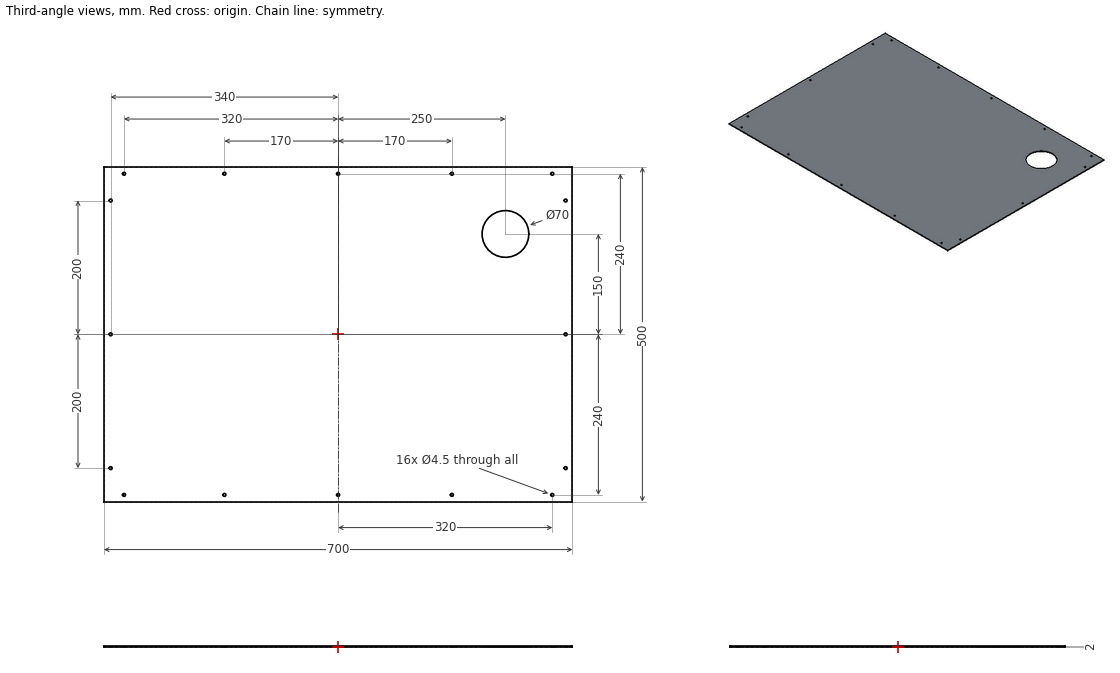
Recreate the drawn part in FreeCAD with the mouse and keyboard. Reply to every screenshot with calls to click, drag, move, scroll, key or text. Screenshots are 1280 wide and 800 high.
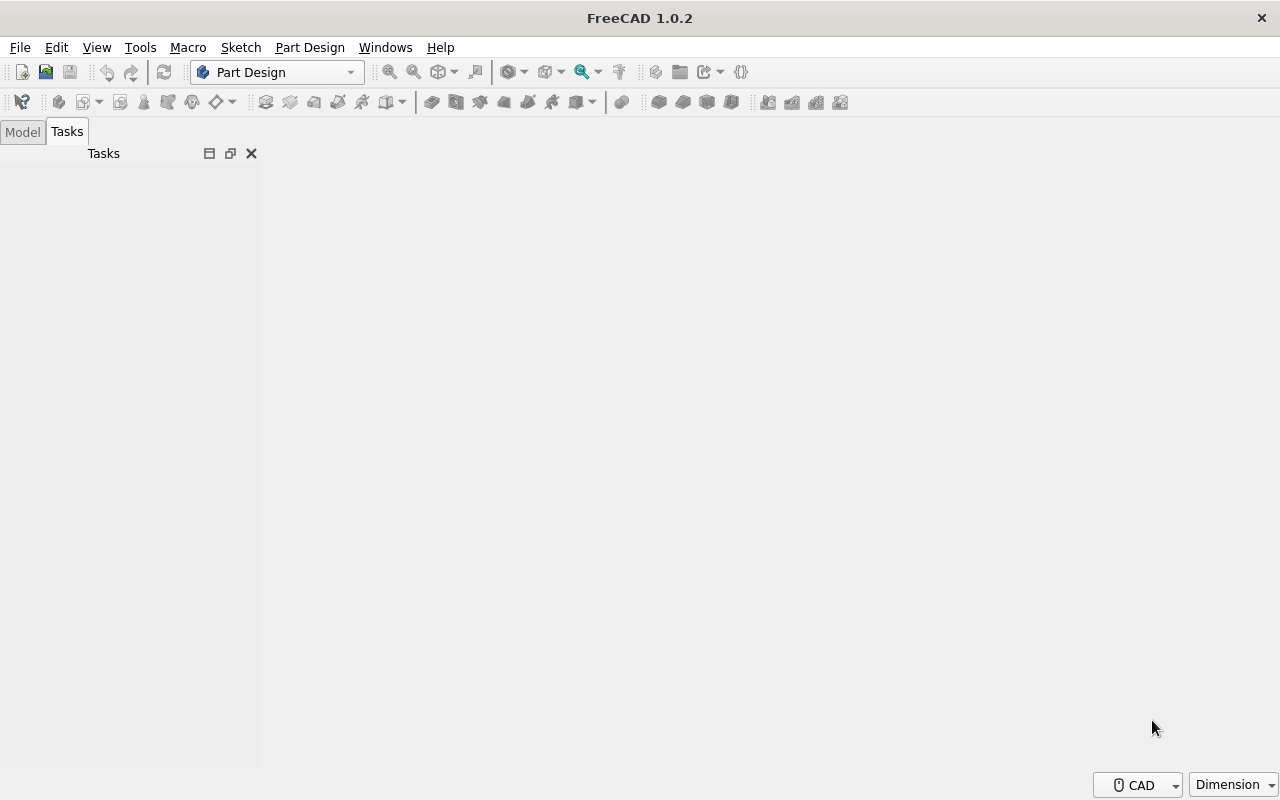
key(ctrl+n)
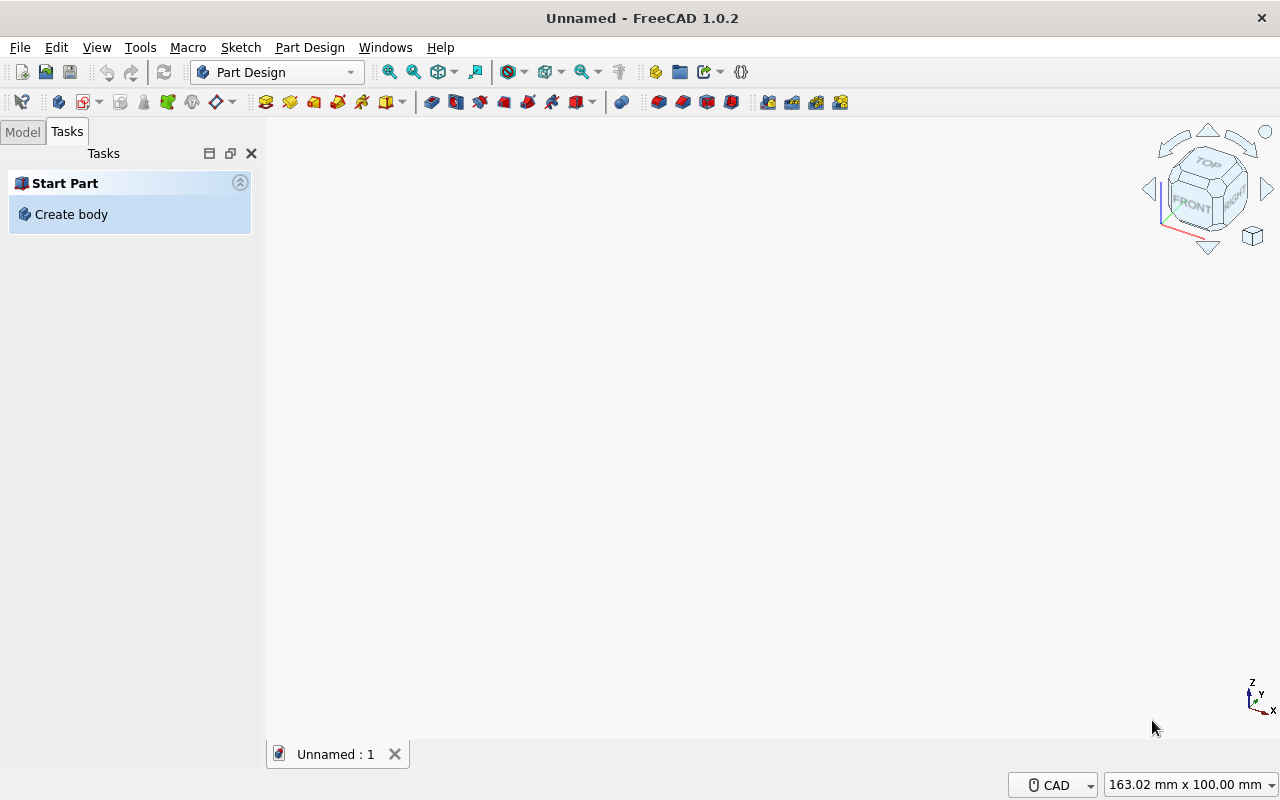
click(84, 102)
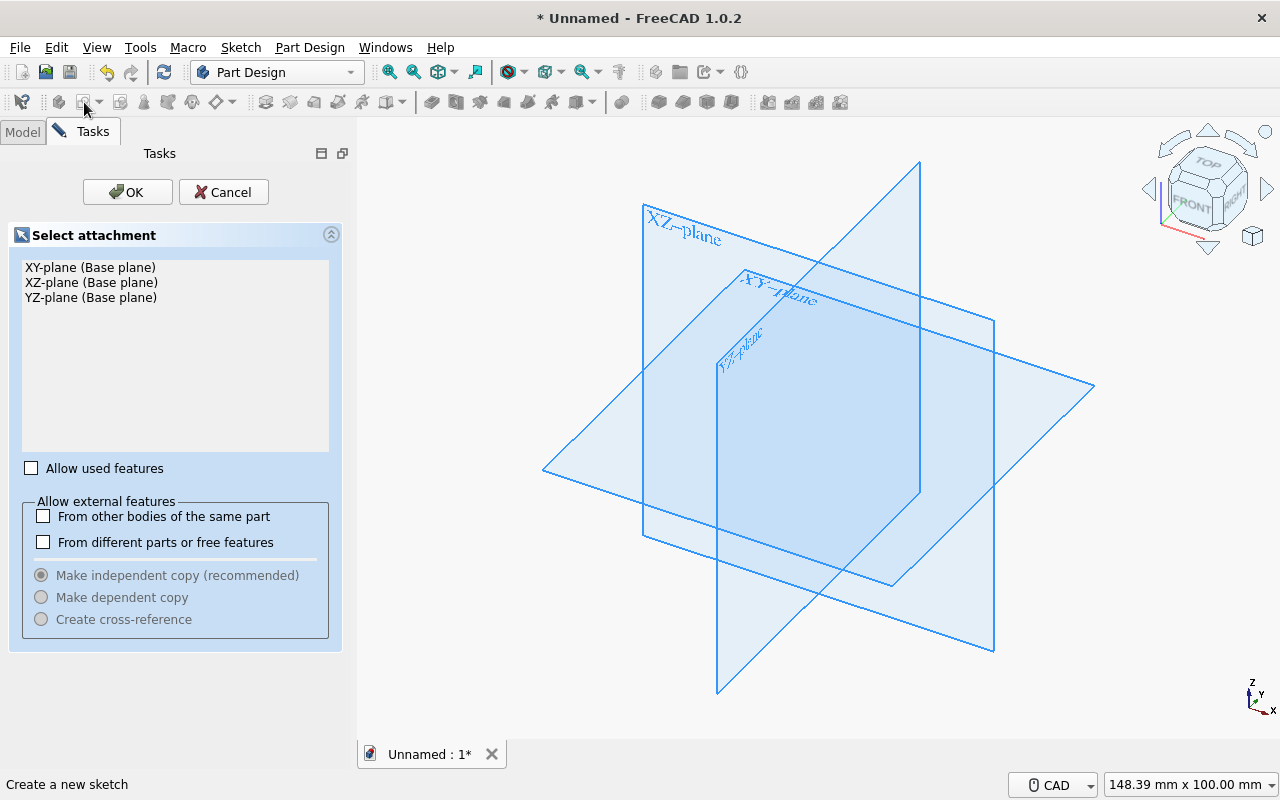
click(82, 268)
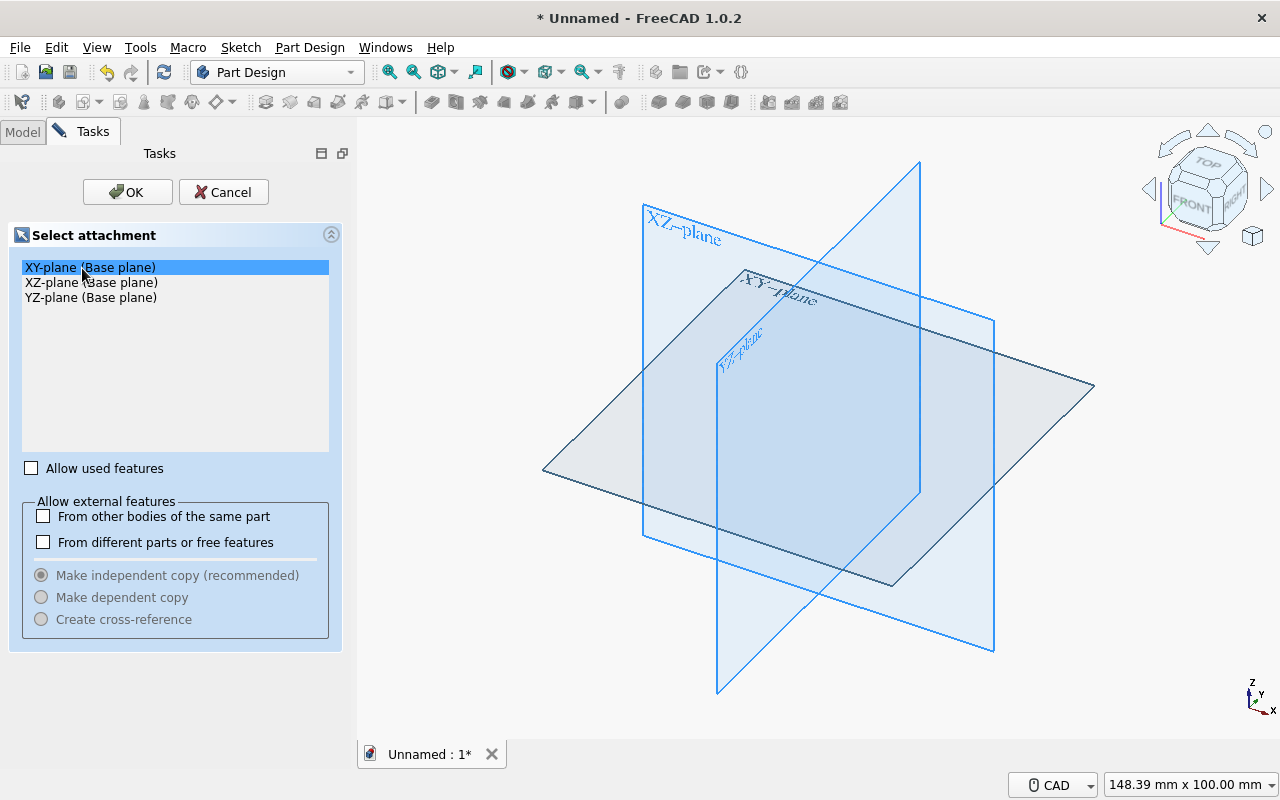
click(128, 192)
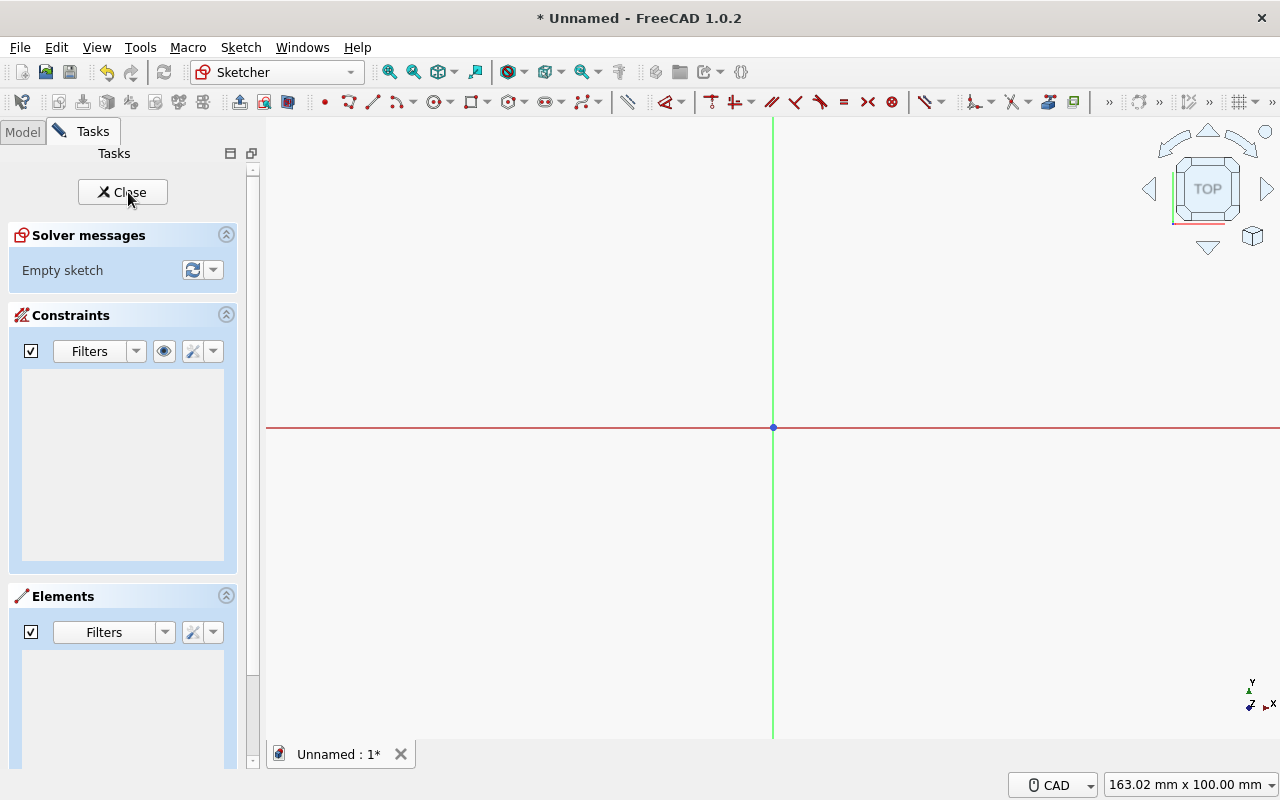
scroll(694, 428, down, 10)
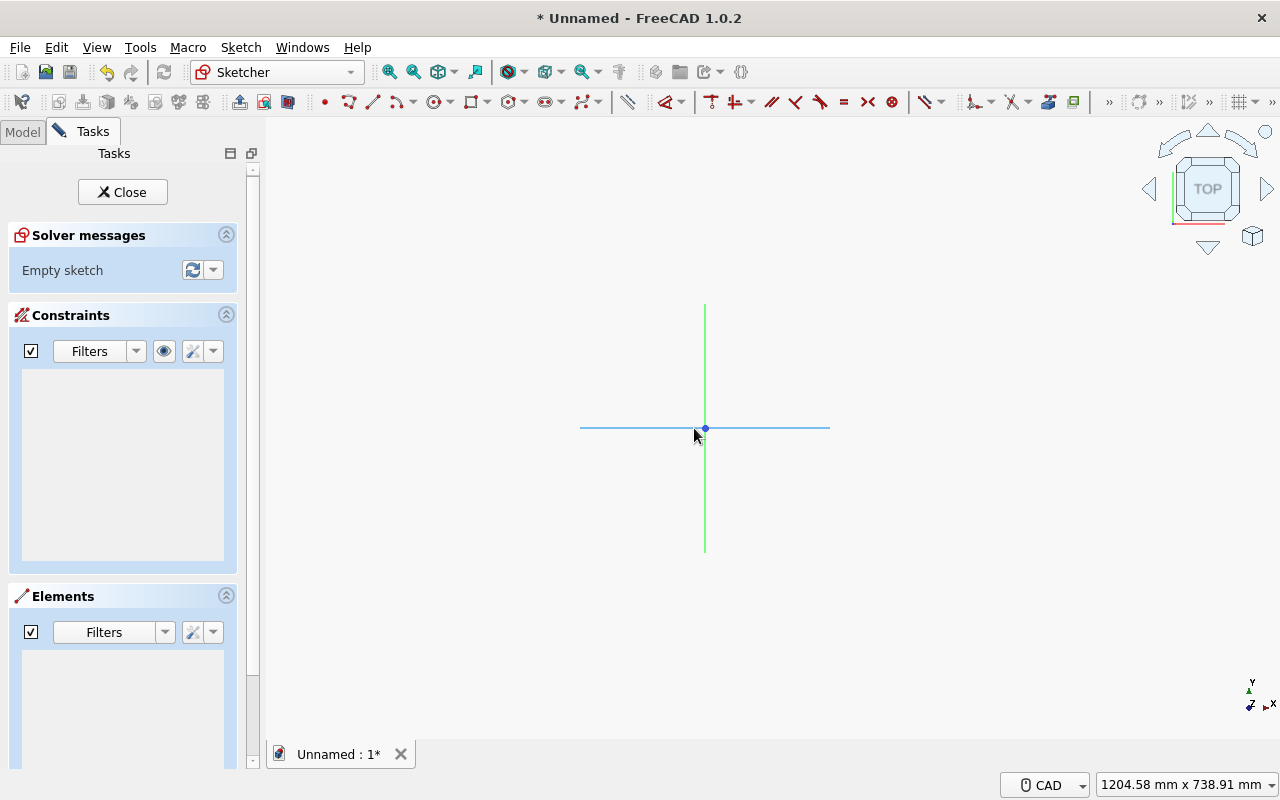
key(g)
key(v)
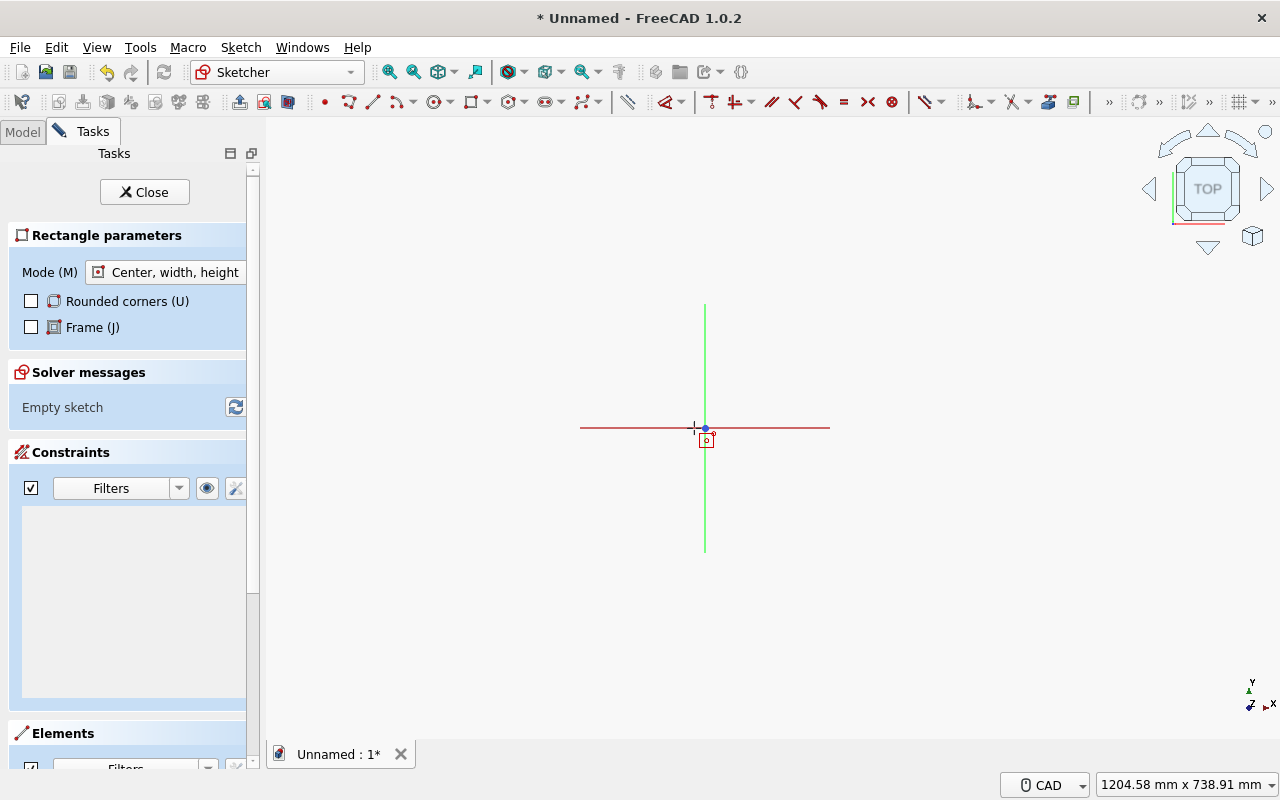
click(705, 428)
move(1000, 218)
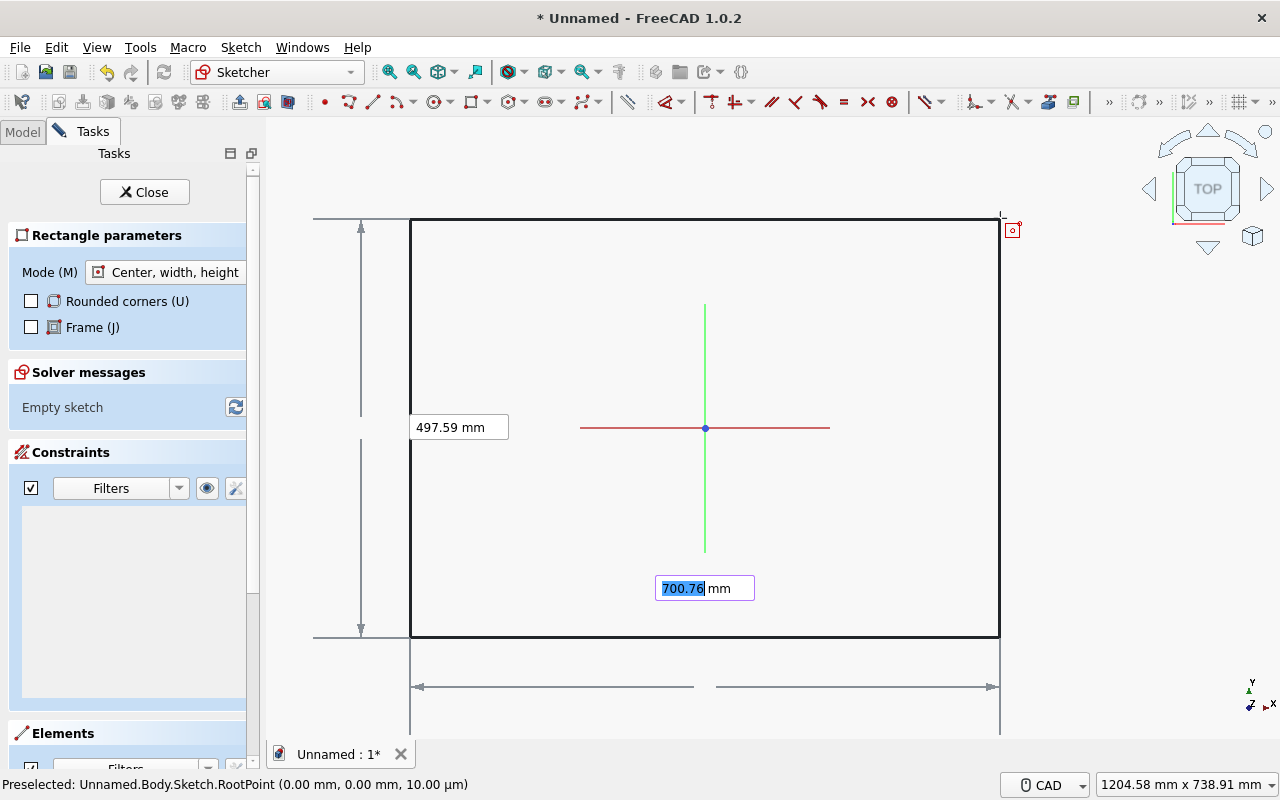
text(700)
key(Tab)
text(500)
key(Return)
key(Escape)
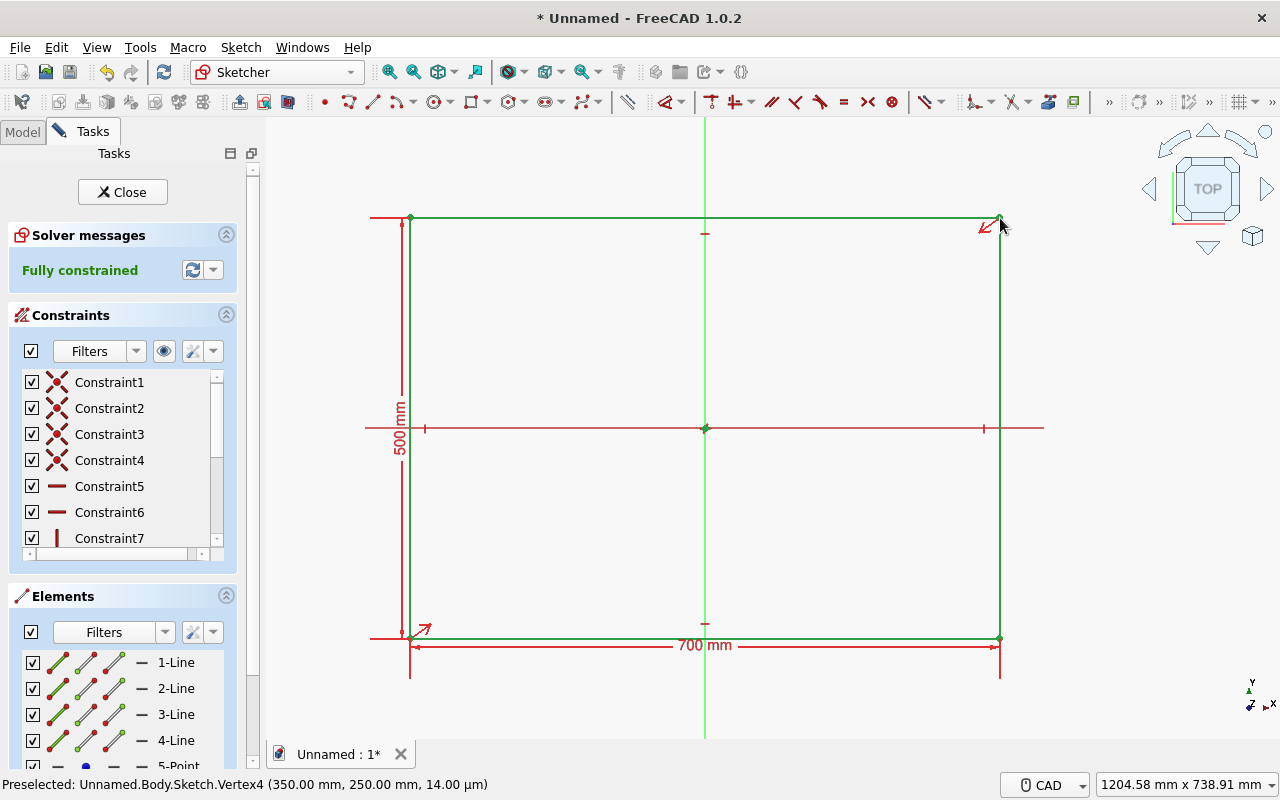
click(123, 192)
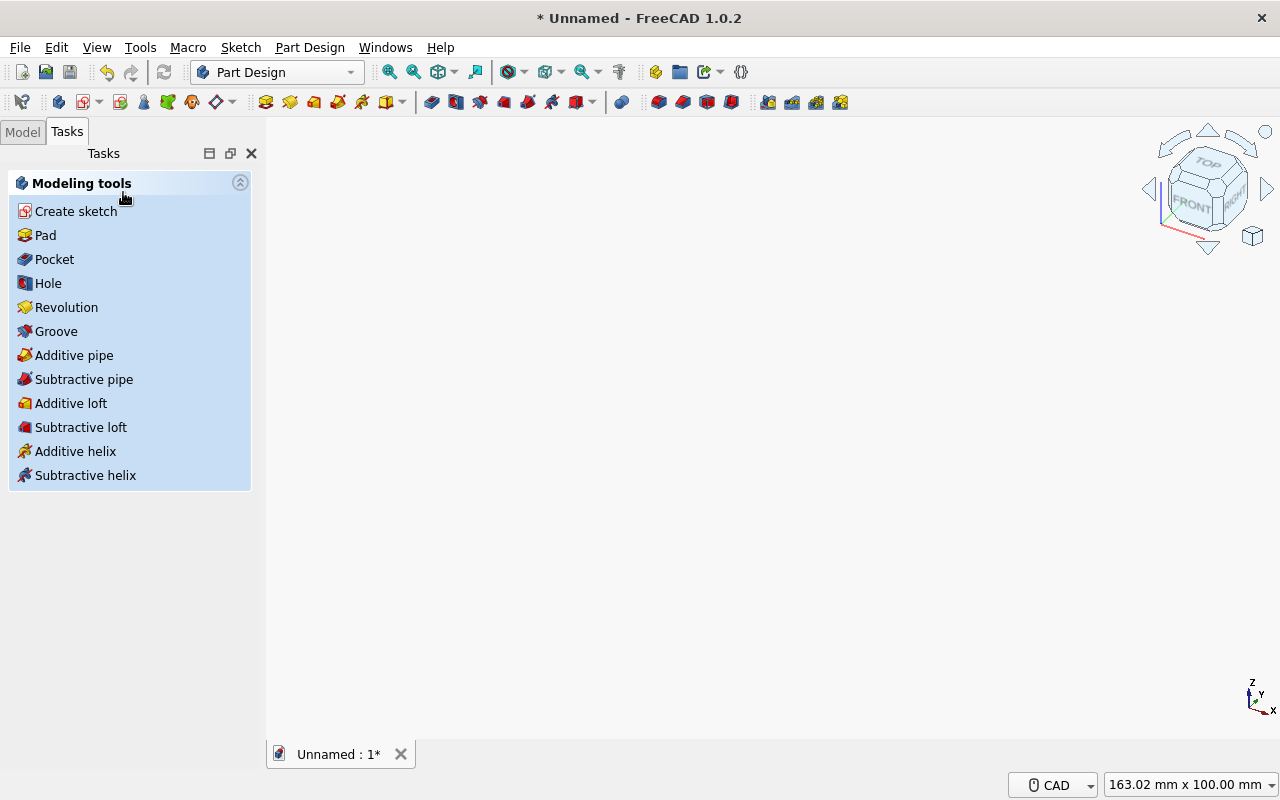
click(266, 102)